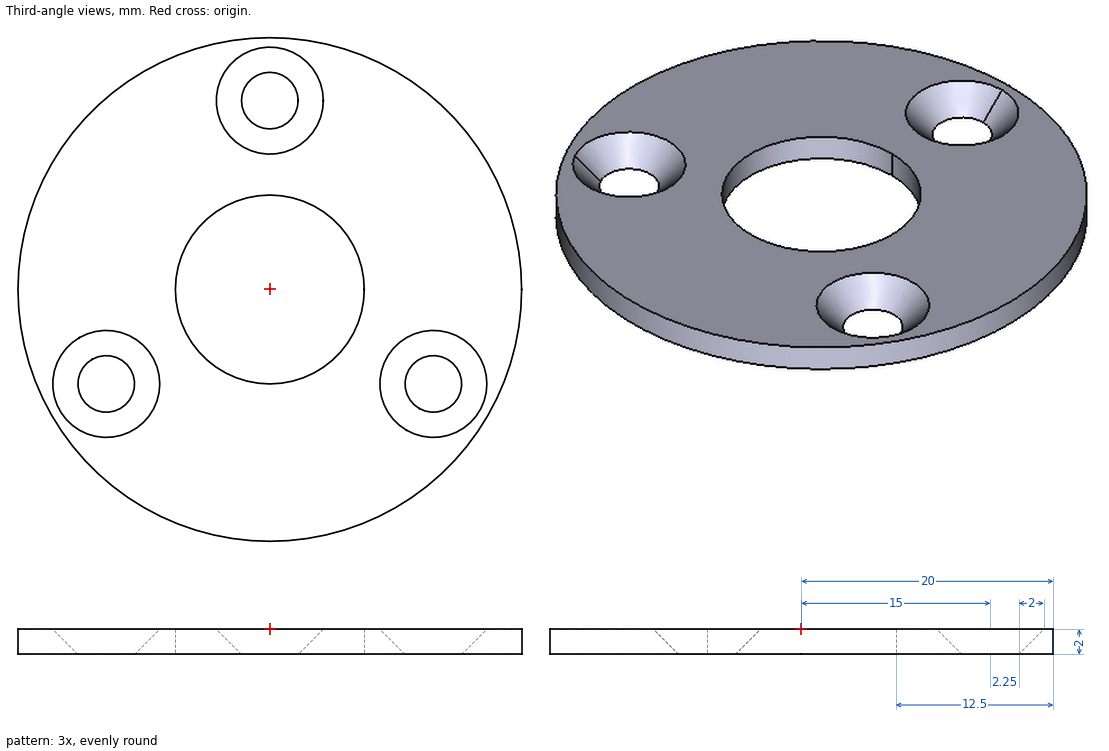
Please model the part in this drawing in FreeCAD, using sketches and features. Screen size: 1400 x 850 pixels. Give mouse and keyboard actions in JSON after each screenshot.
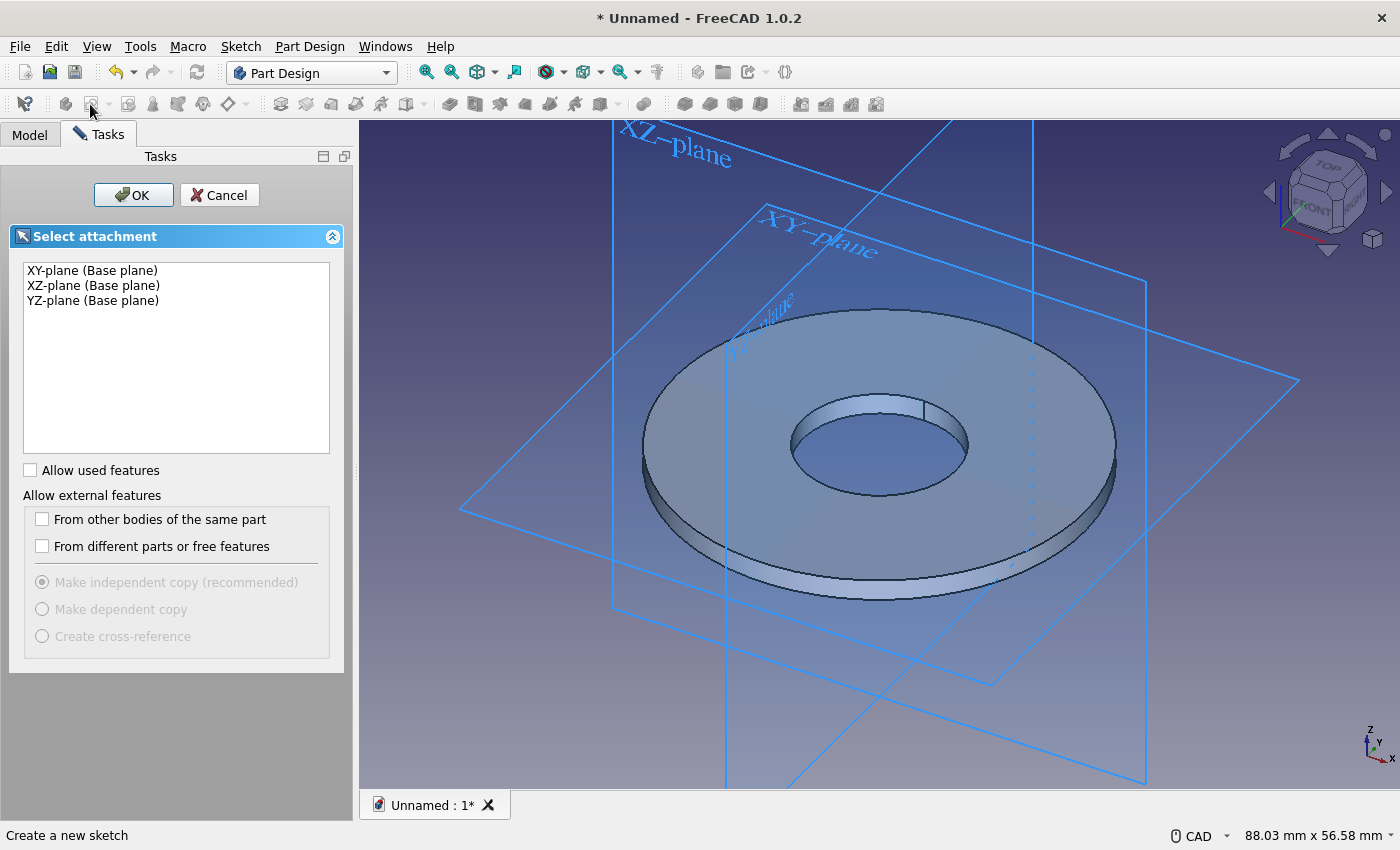
{"action": "left_click", "coordinate": [84, 300]}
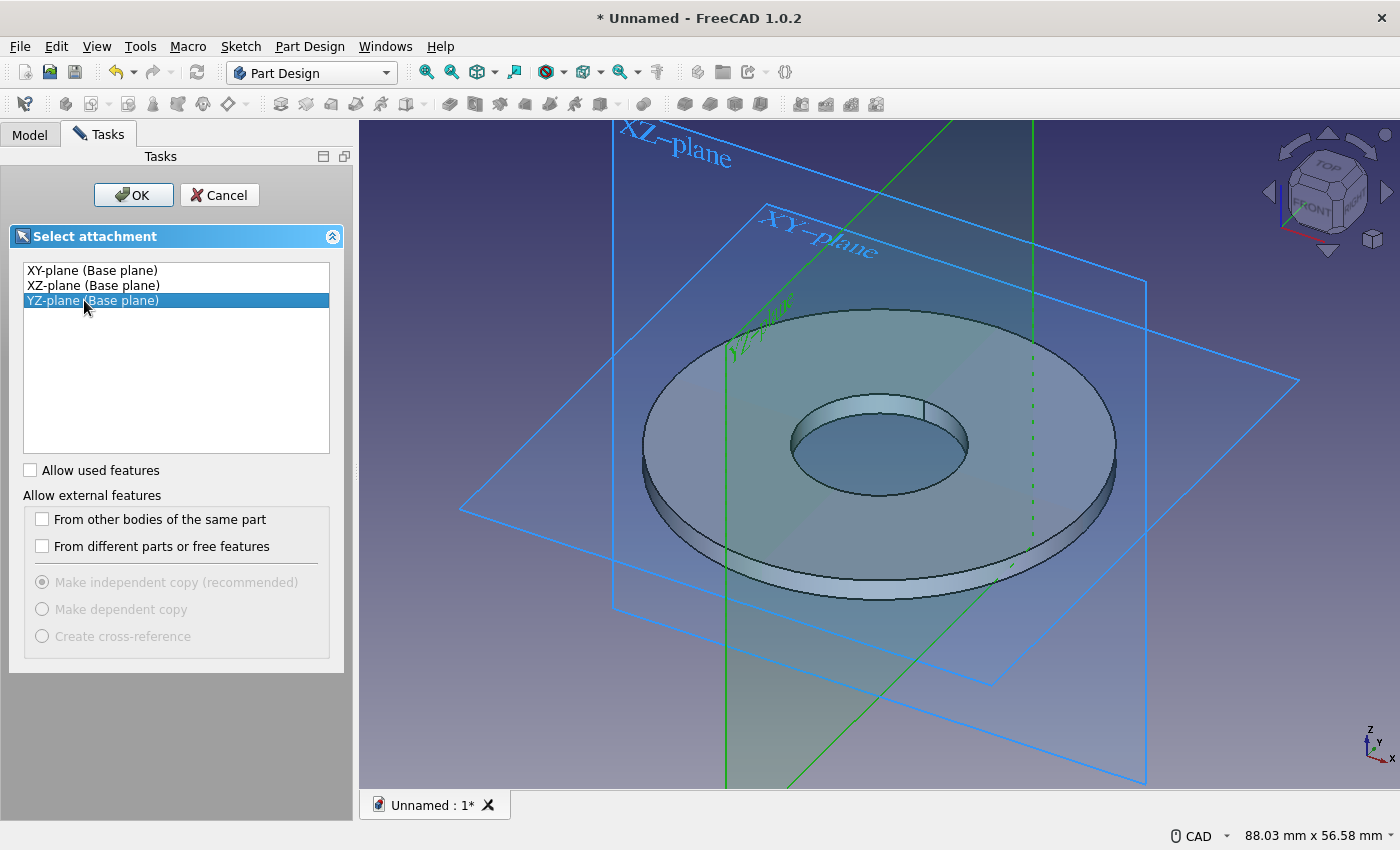
{"action": "left_click", "coordinate": [134, 195]}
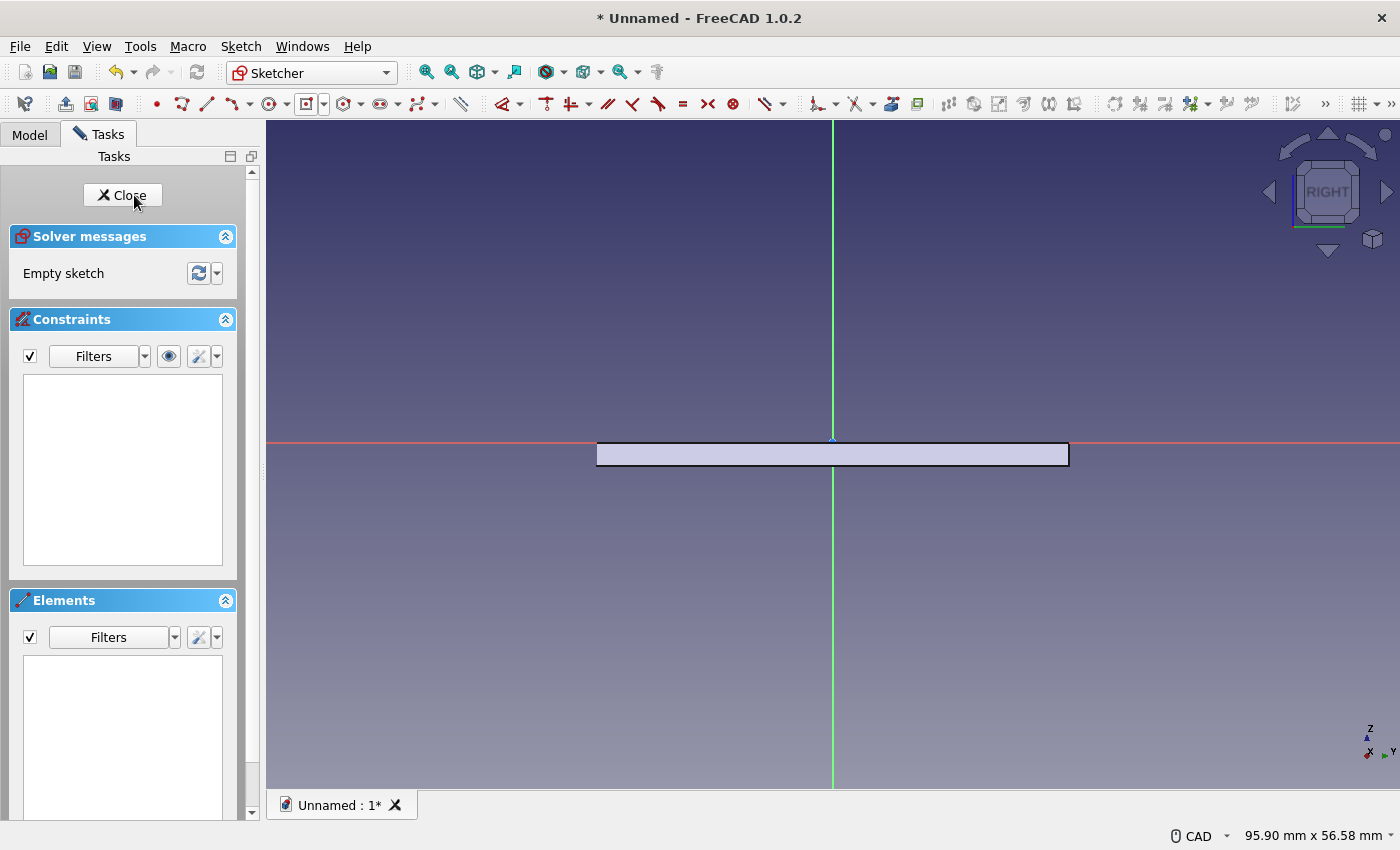
{"action": "left_click", "coordinate": [116, 104]}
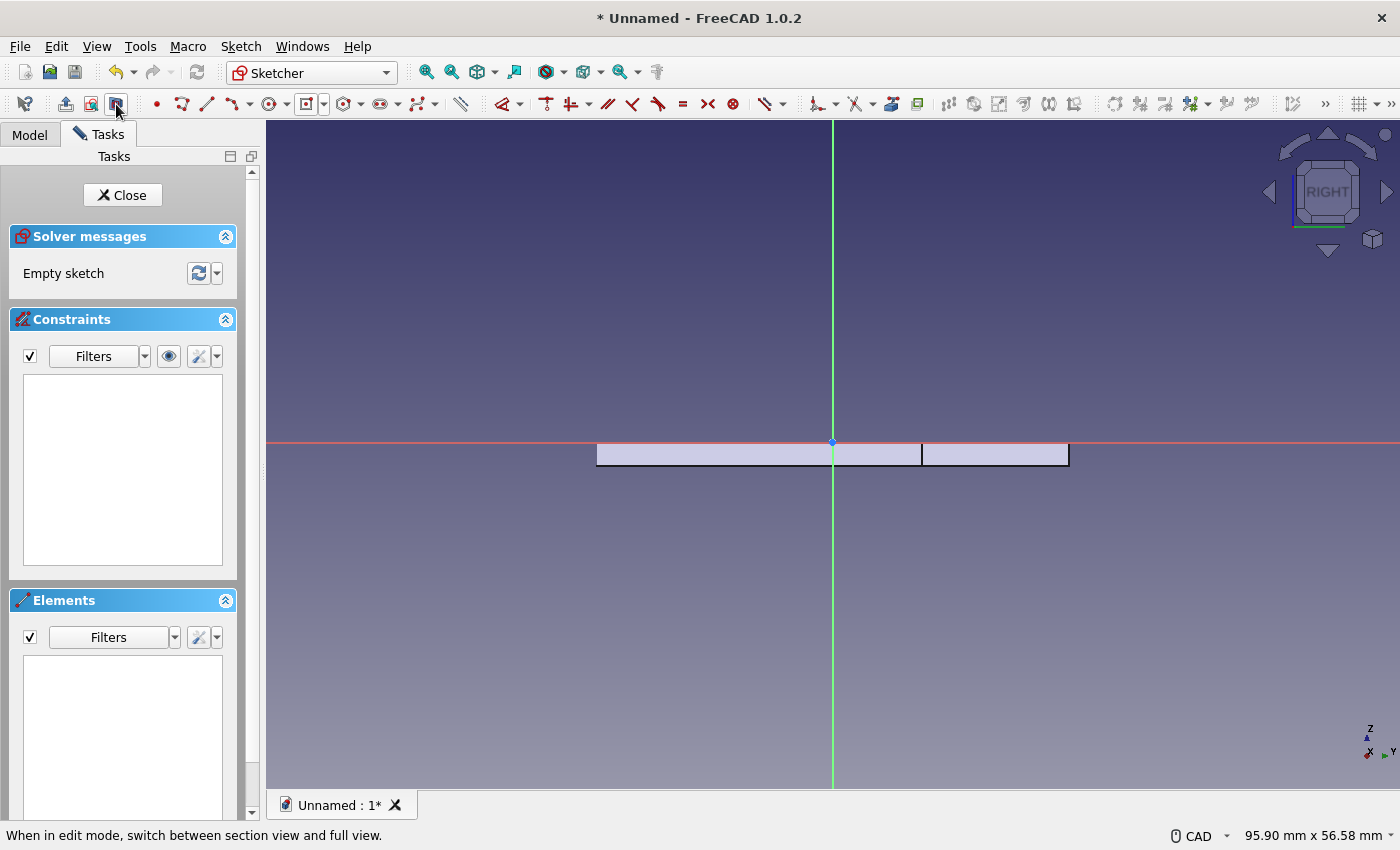
{"action": "scroll", "coordinate": [1057, 460], "scroll_direction": "up", "scroll_amount": 13}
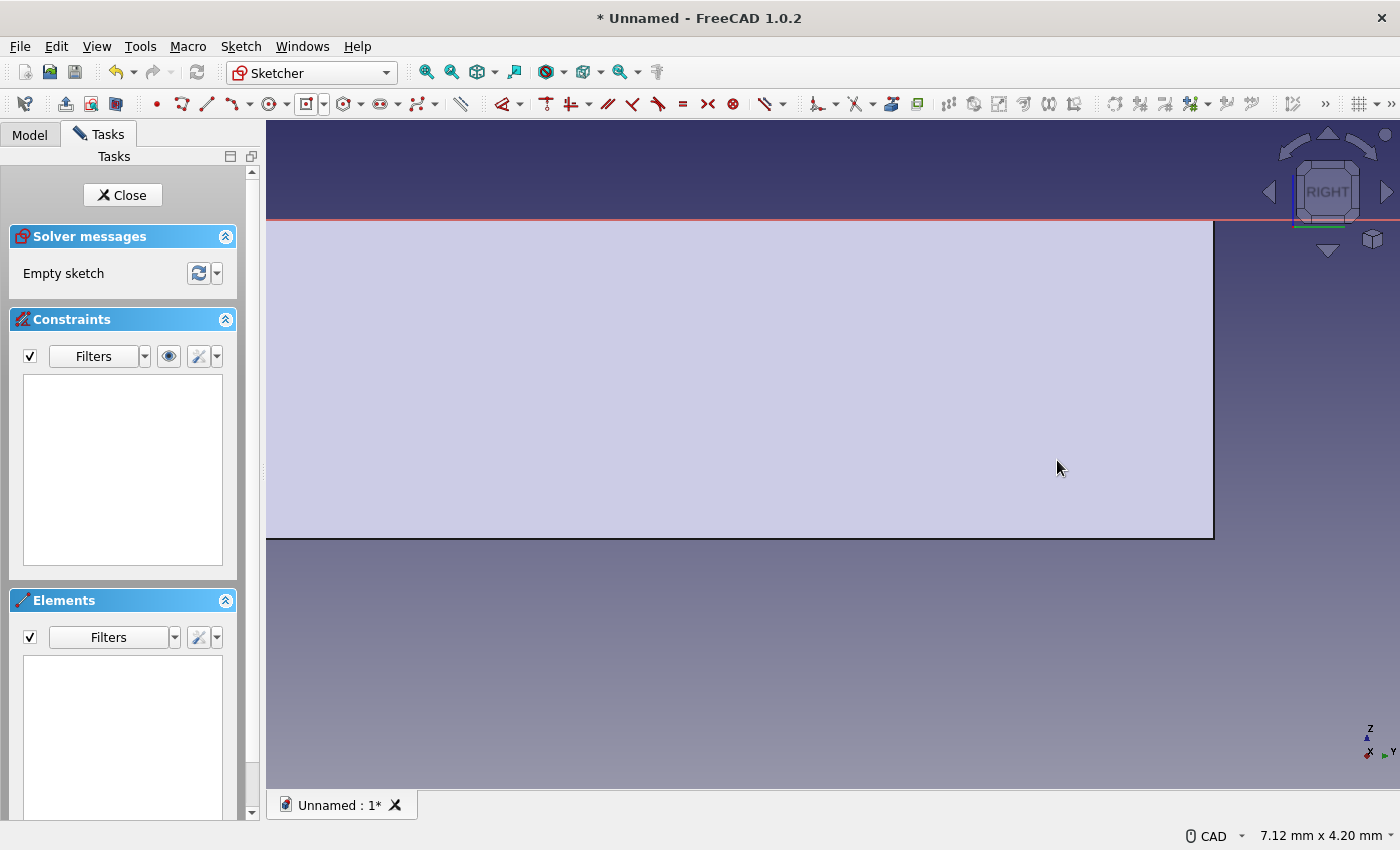
{"action": "left_click", "coordinate": [182, 104]}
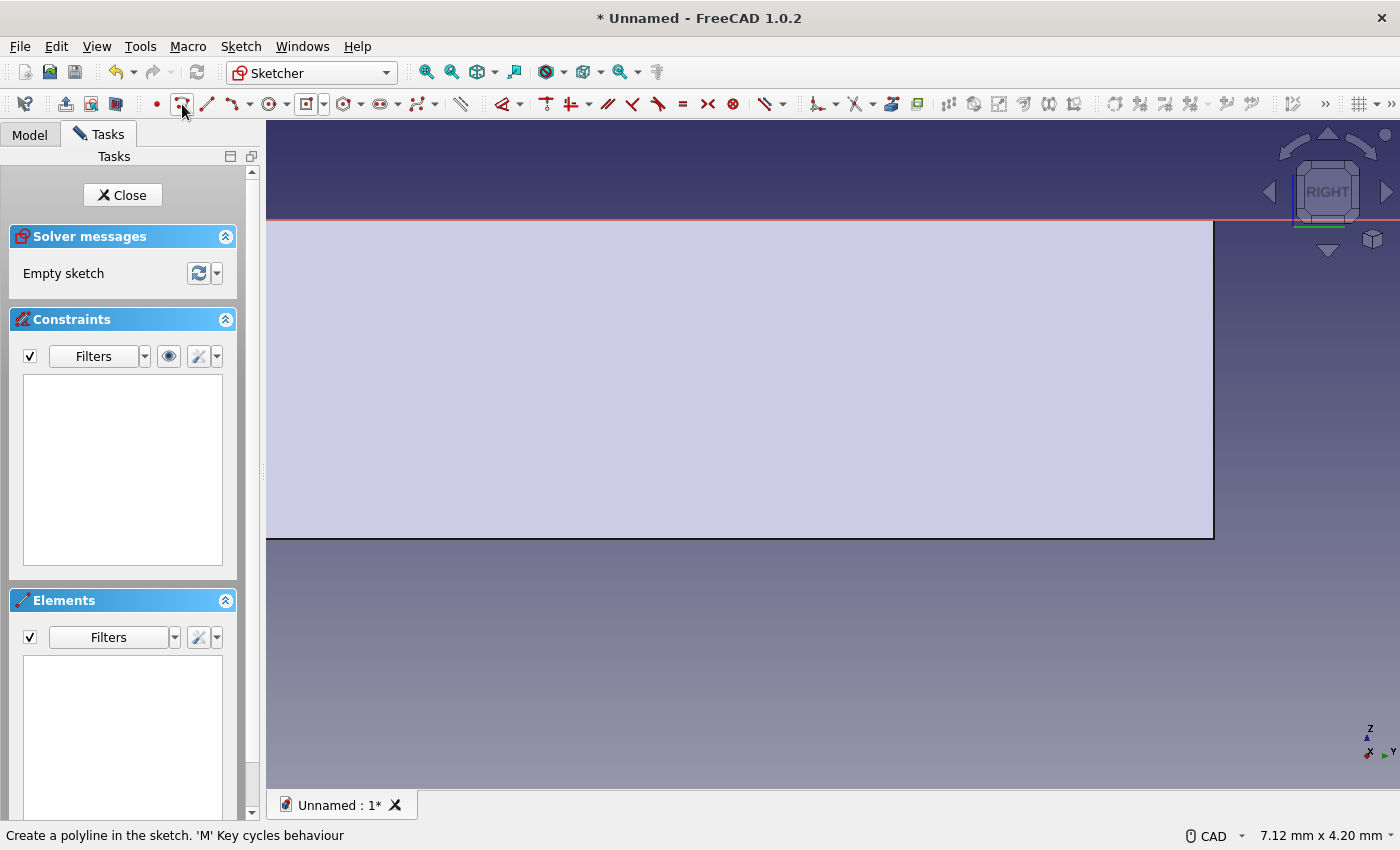
{"action": "left_click", "coordinate": [418, 220]}
{"action": "left_click", "coordinate": [418, 539]}
{"action": "left_click", "coordinate": [777, 539]}
{"action": "left_click", "coordinate": [1095, 229]}
{"action": "left_click", "coordinate": [418, 220]}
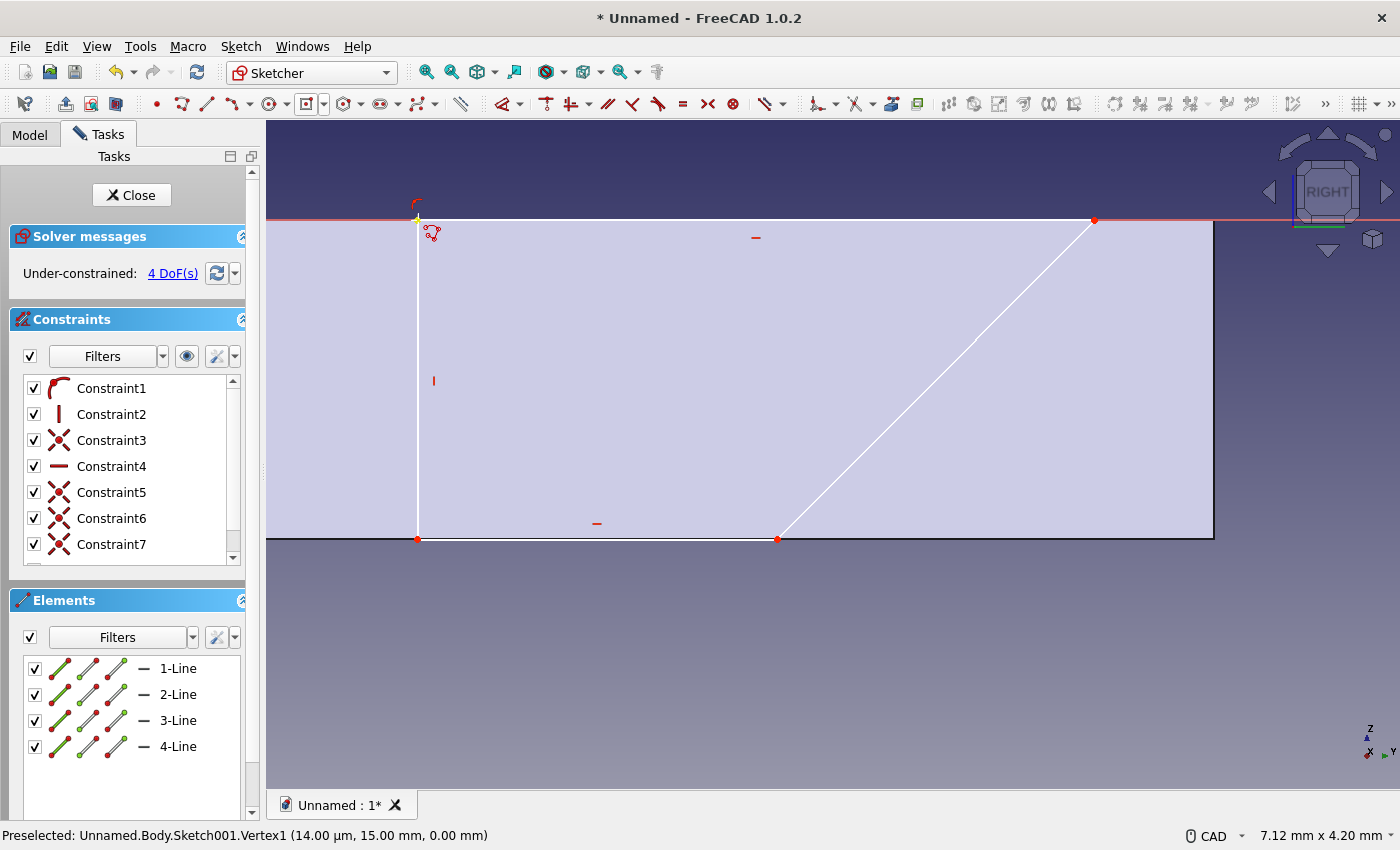
{"action": "left_click", "coordinate": [207, 104]}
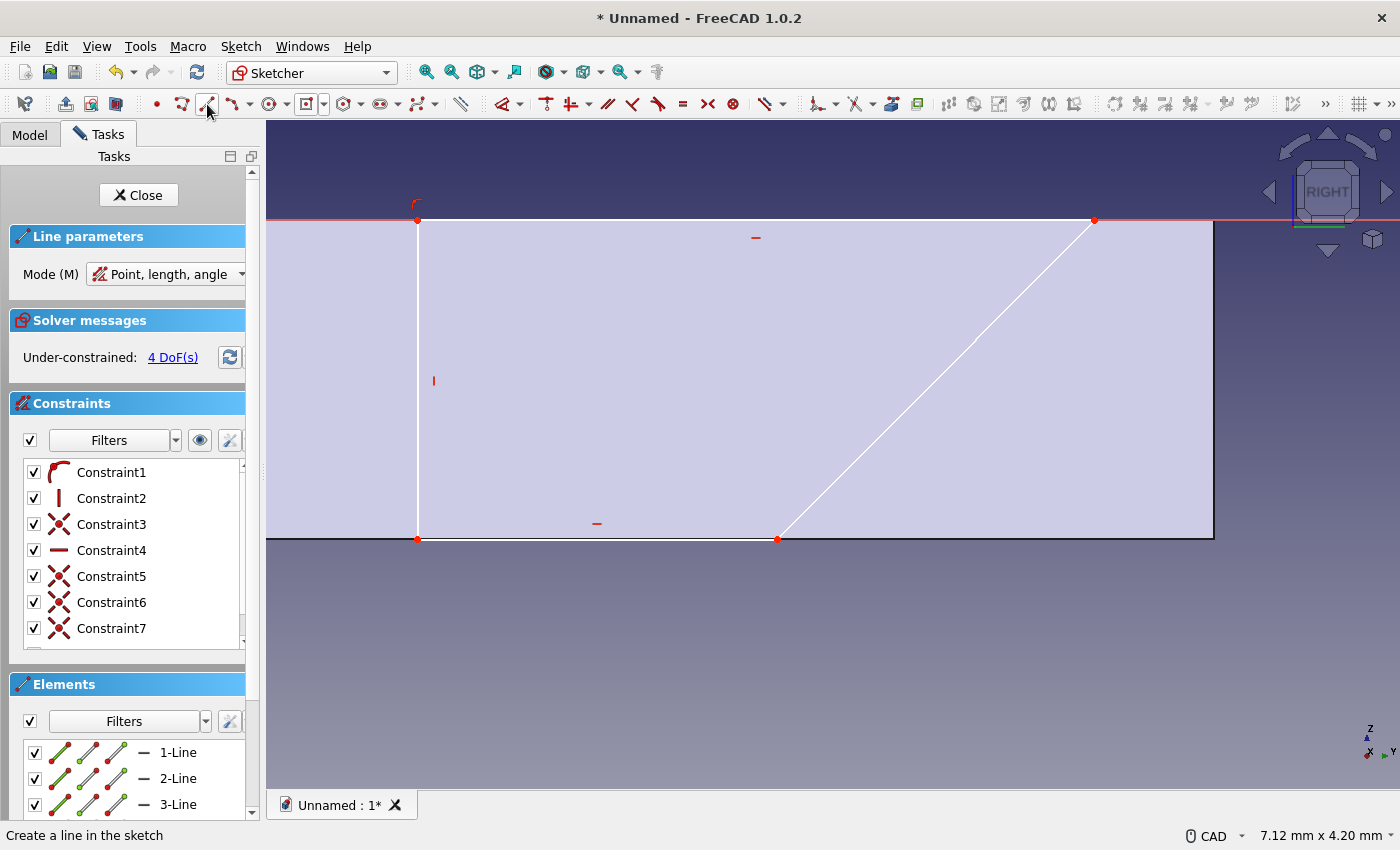
{"action": "left_click", "coordinate": [418, 571]}
{"action": "left_click", "coordinate": [418, 666]}
{"action": "key", "text": "Escape"}